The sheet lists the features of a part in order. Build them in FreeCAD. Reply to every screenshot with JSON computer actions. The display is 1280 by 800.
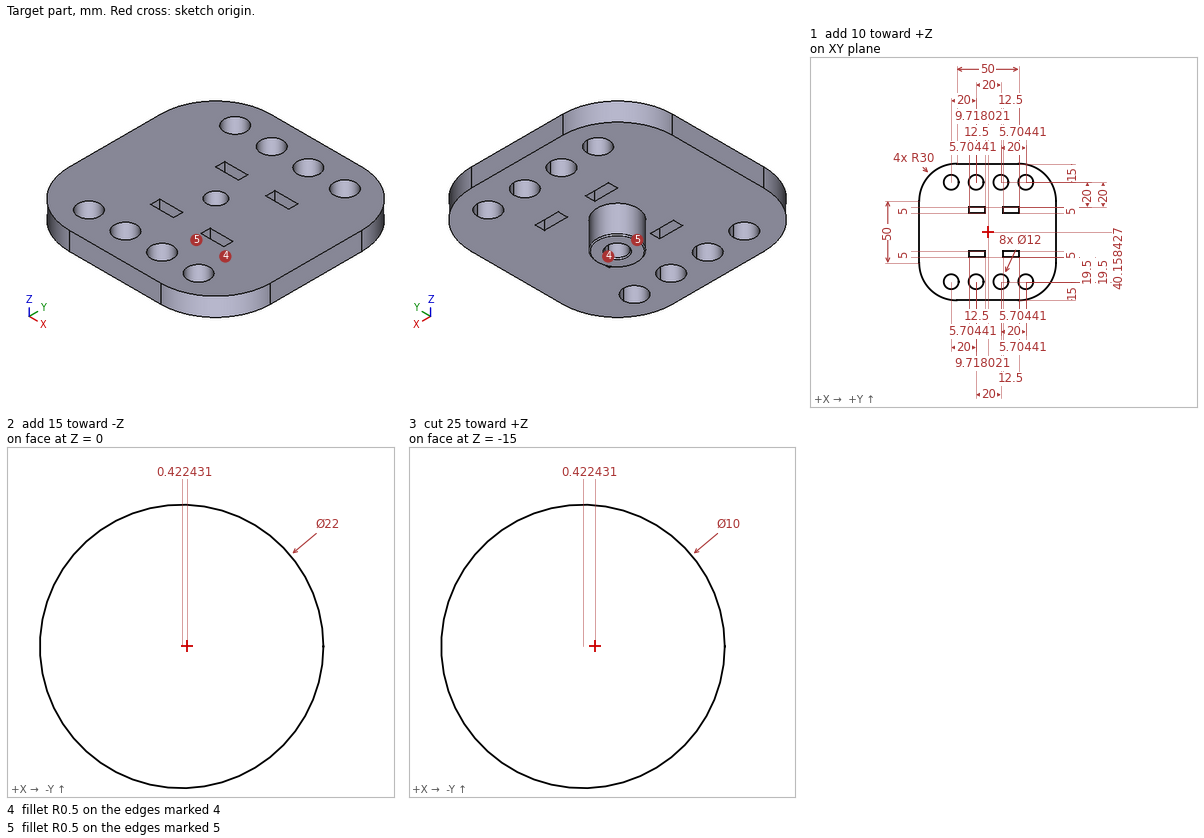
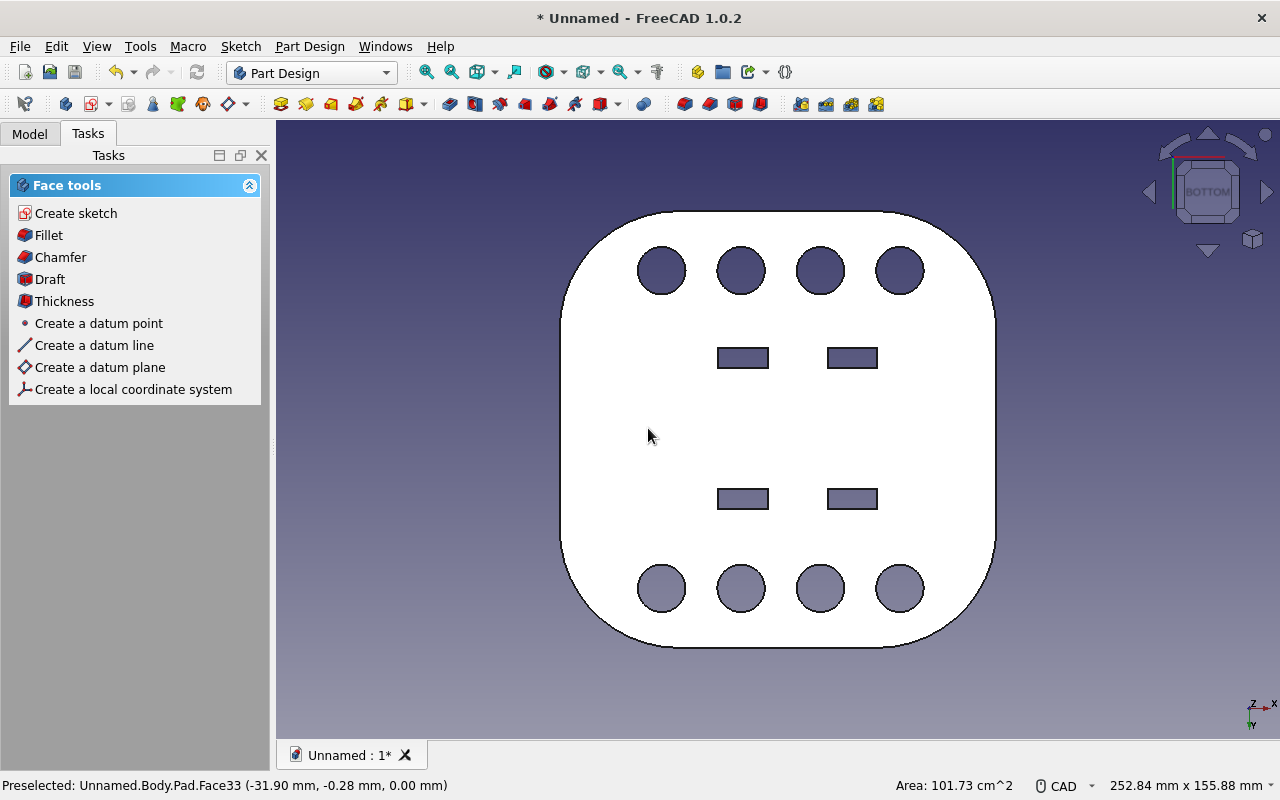
{"action": "left_click", "coordinate": [90, 104]}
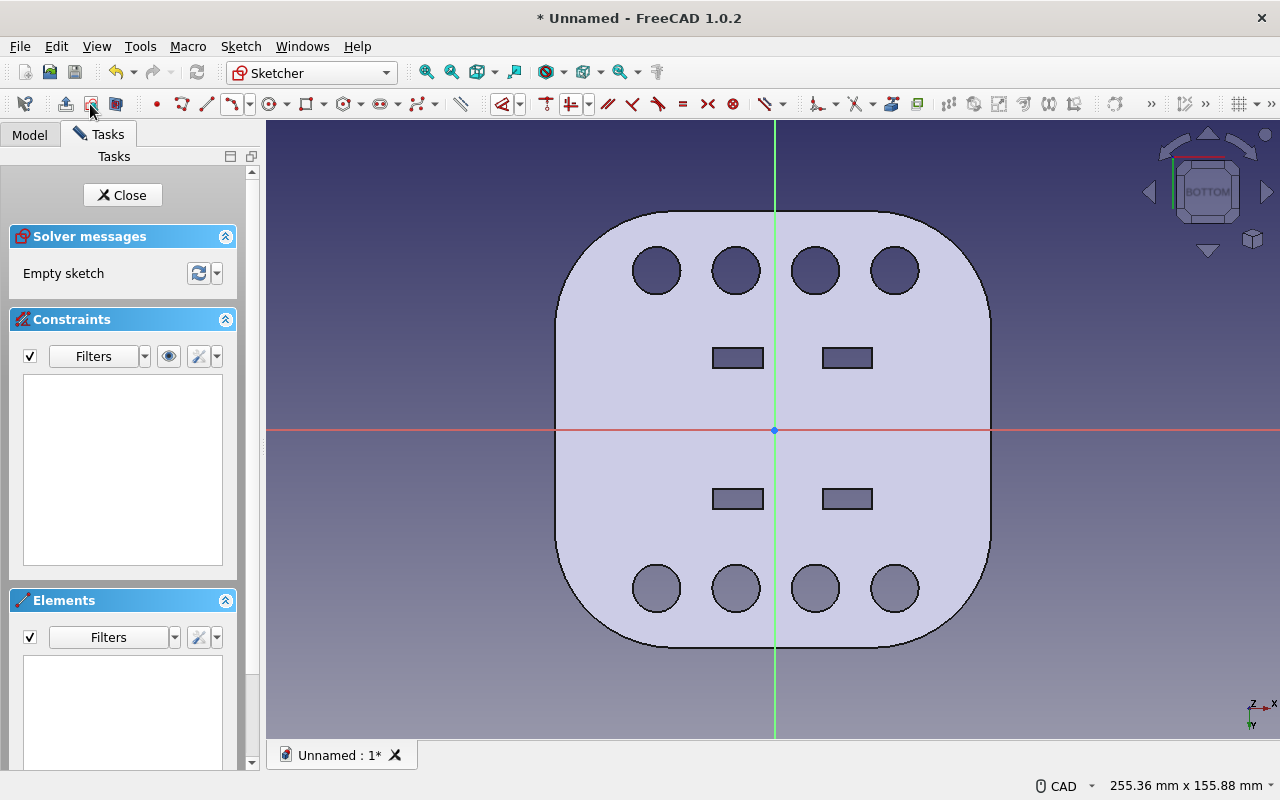
{"action": "scroll", "coordinate": [790, 430], "scroll_direction": "up", "scroll_amount": 8}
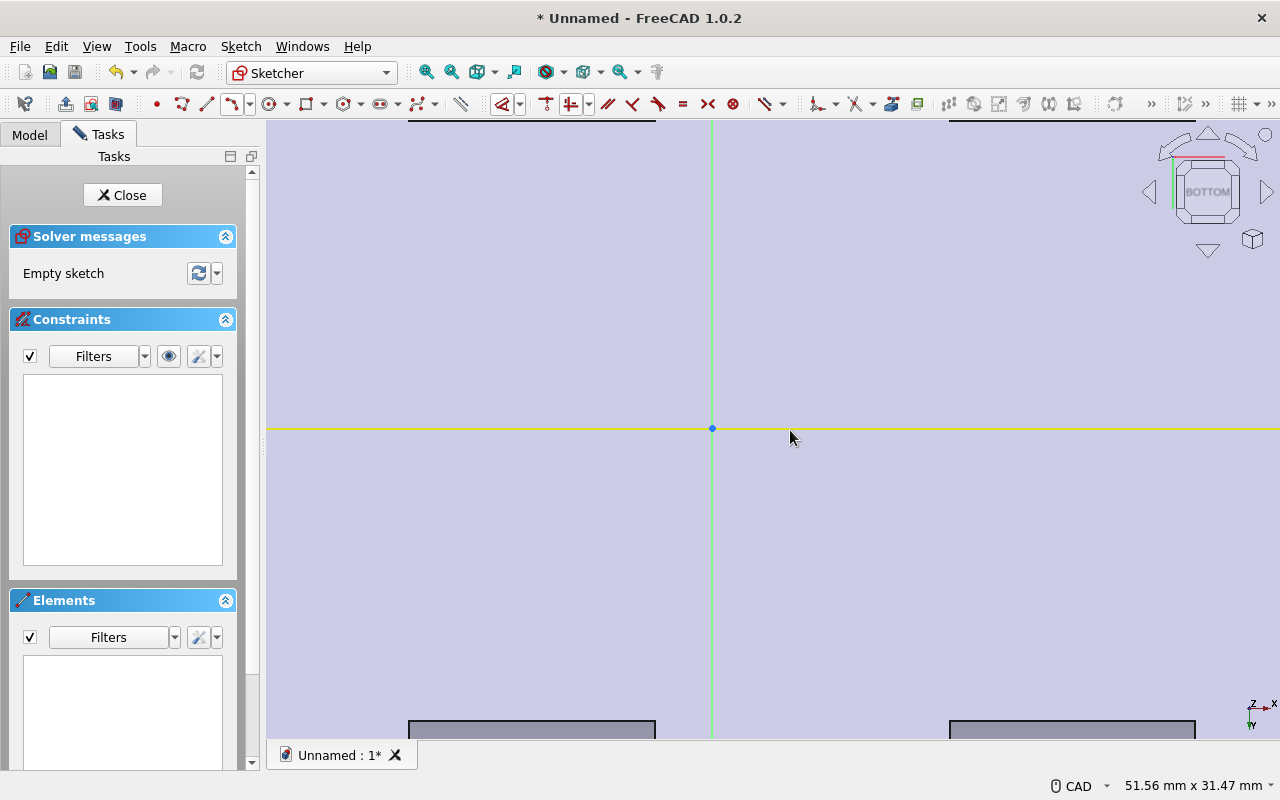
{"action": "left_click", "coordinate": [268, 104]}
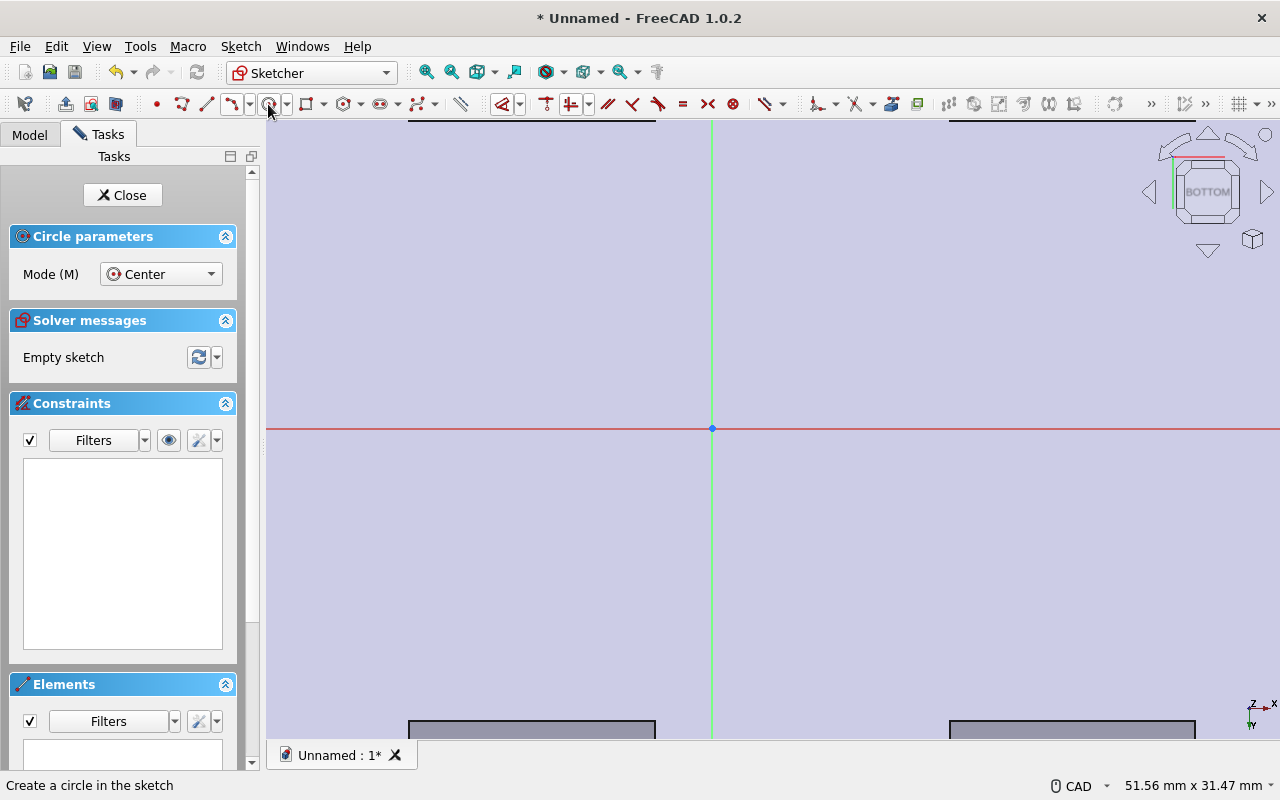
{"action": "scroll", "coordinate": [704, 429], "scroll_direction": "up", "scroll_amount": 4}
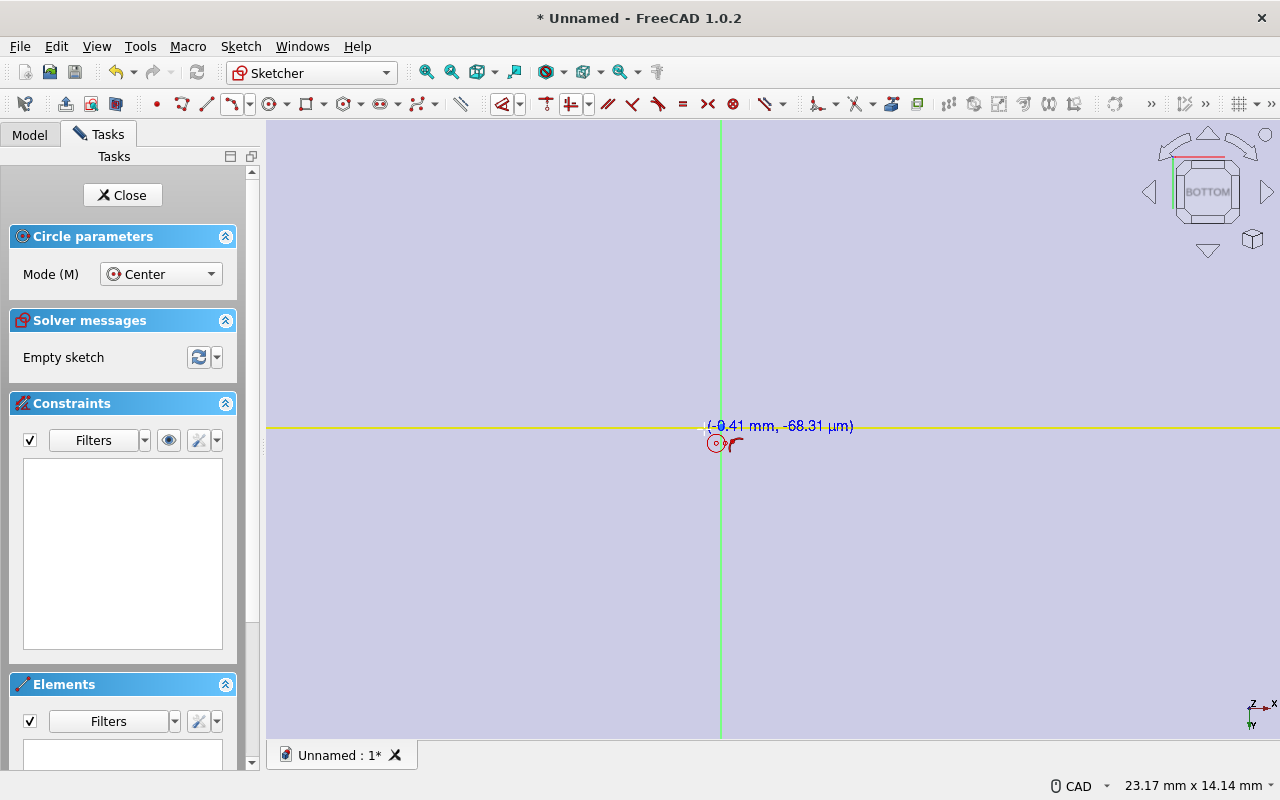
{"action": "left_click", "coordinate": [703, 428]}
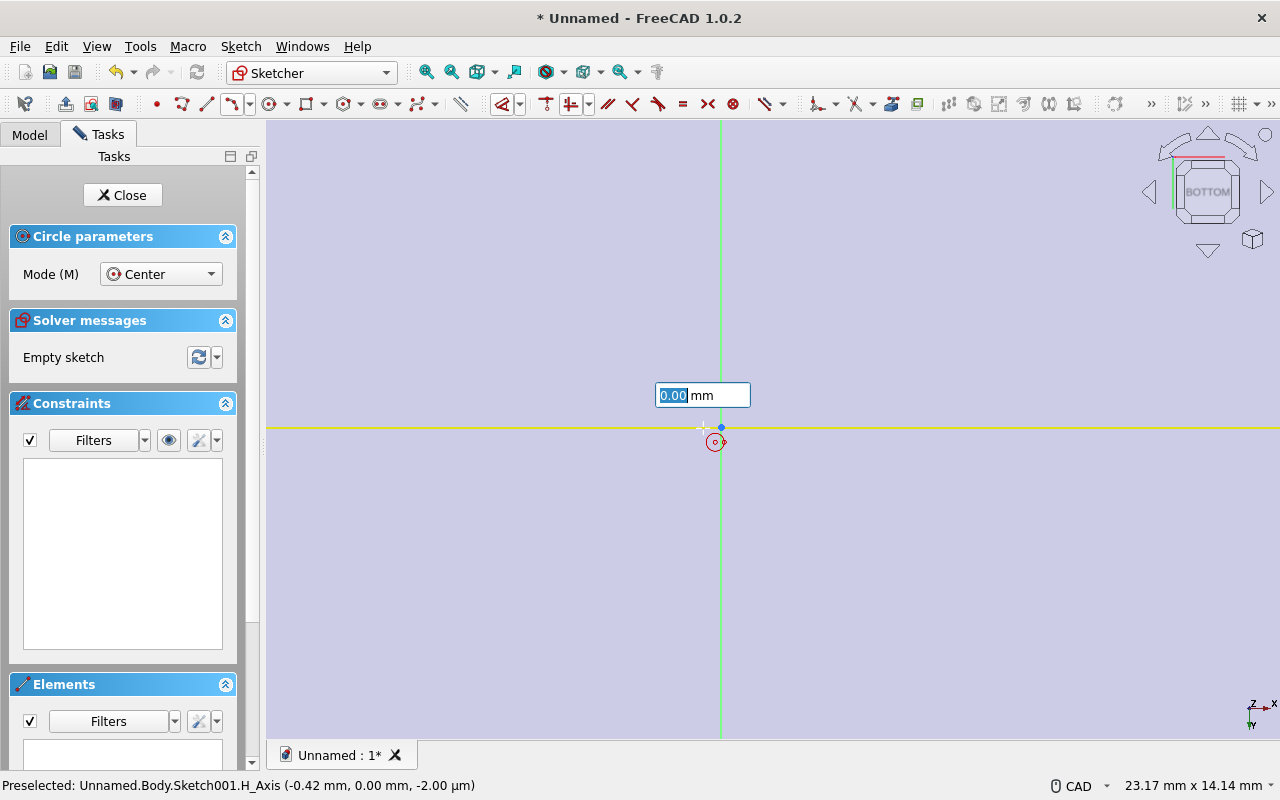
{"action": "scroll", "coordinate": [706, 431], "scroll_direction": "down", "scroll_amount": 4}
{"action": "mouse_move", "coordinate": [858, 277]}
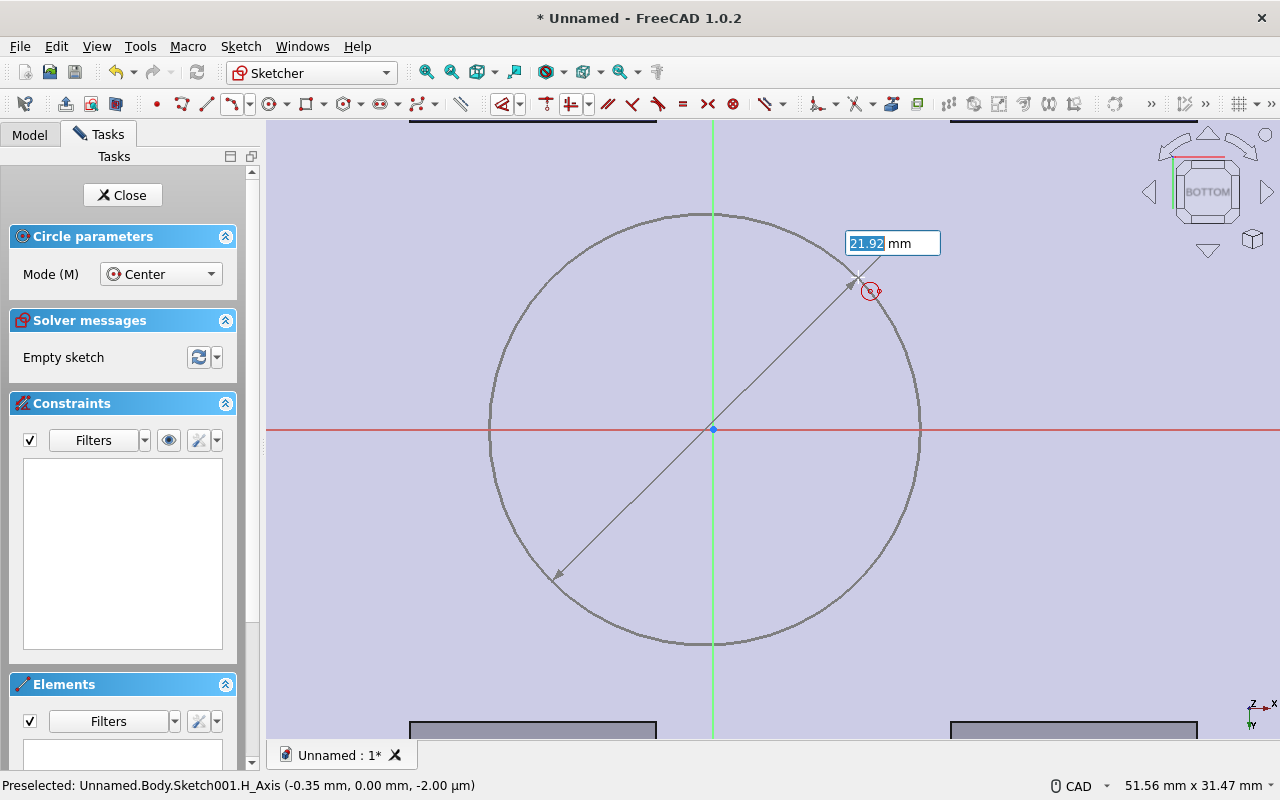
{"action": "type", "text": "22"}
{"action": "key", "text": "Return"}
{"action": "key", "text": "Escape"}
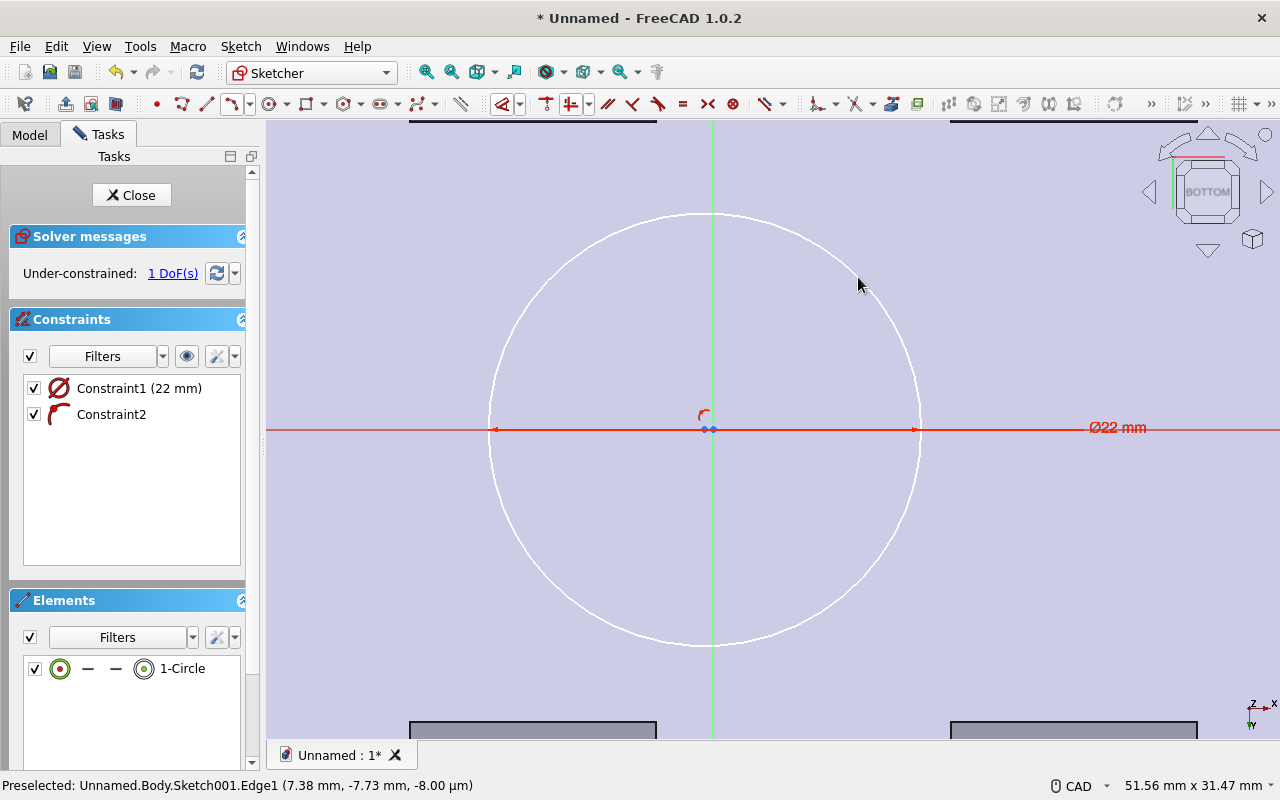
{"action": "scroll", "coordinate": [705, 430], "scroll_direction": "up", "scroll_amount": 8}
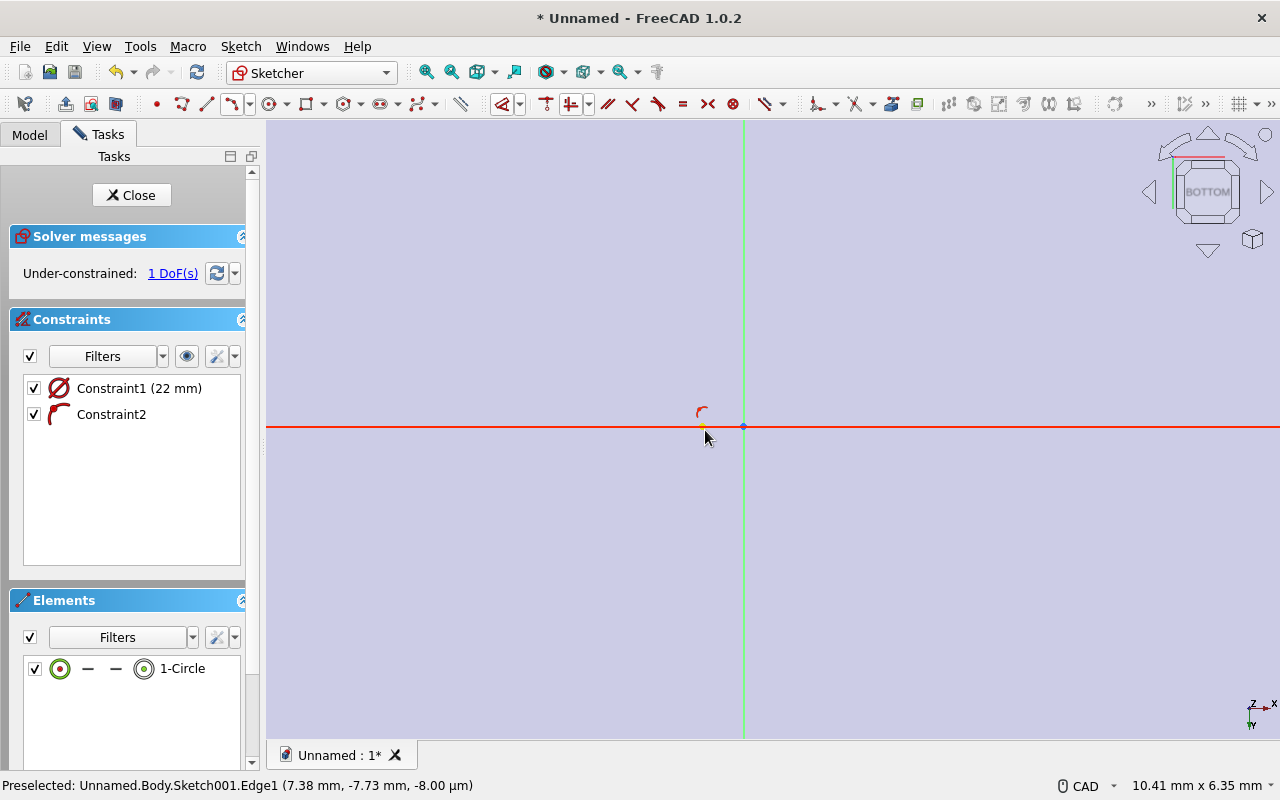
{"action": "left_click", "coordinate": [703, 427]}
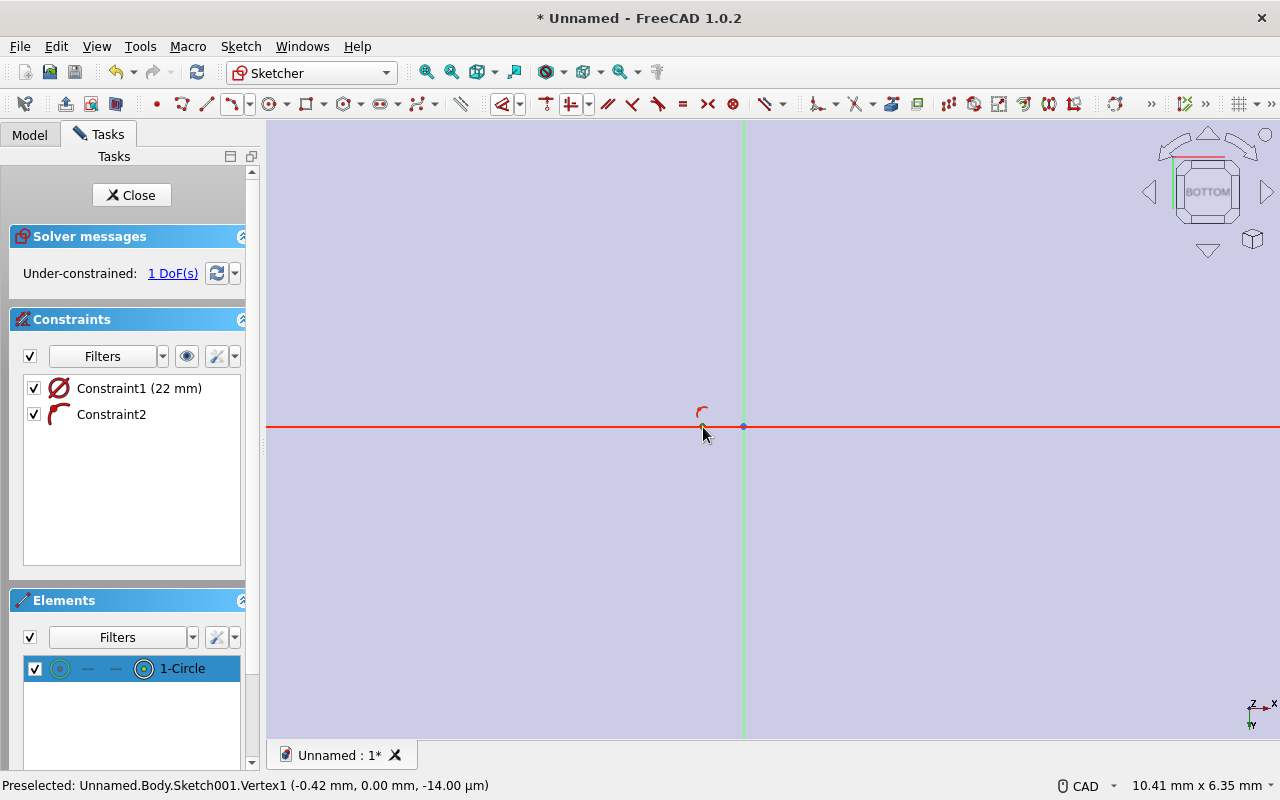
{"action": "left_click", "coordinate": [520, 104]}